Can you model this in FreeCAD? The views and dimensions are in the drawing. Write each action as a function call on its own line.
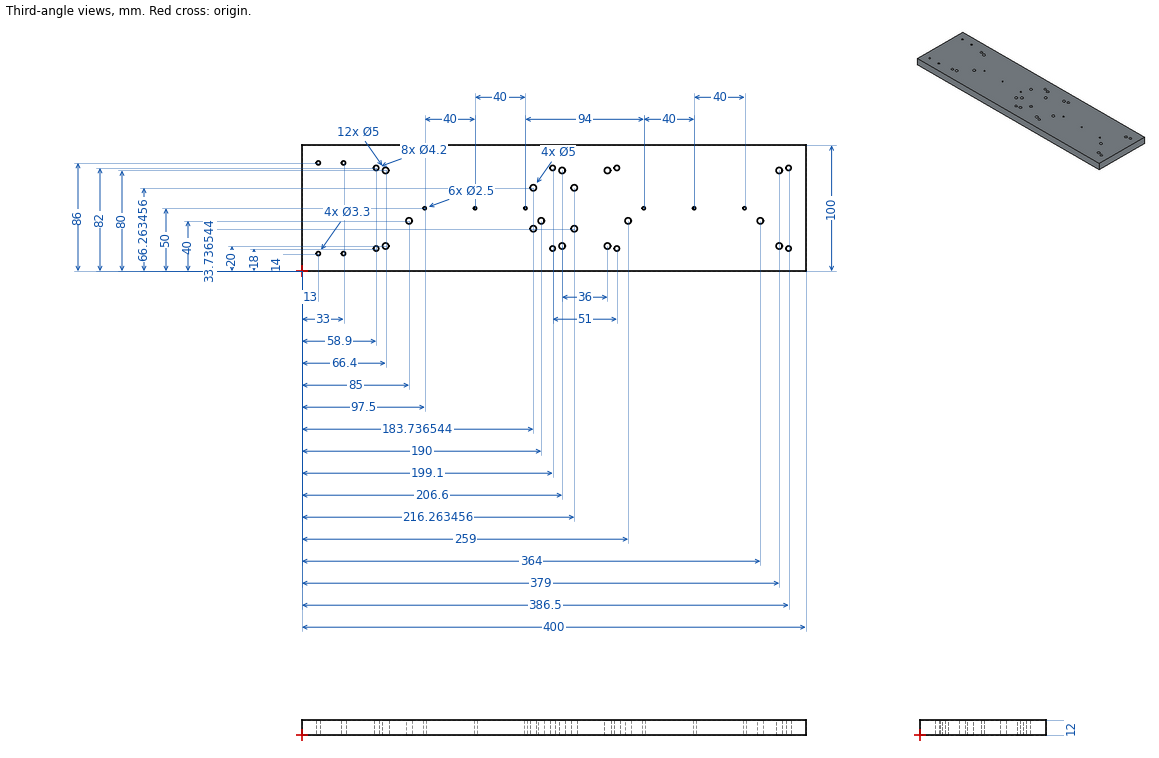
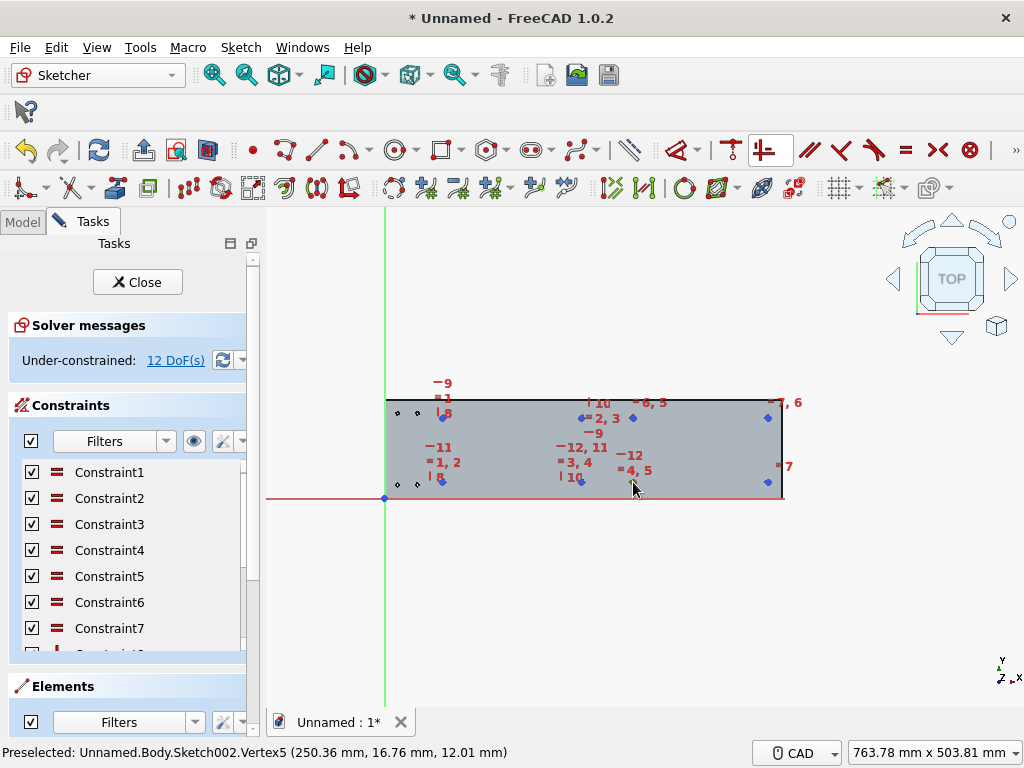
click(633, 418)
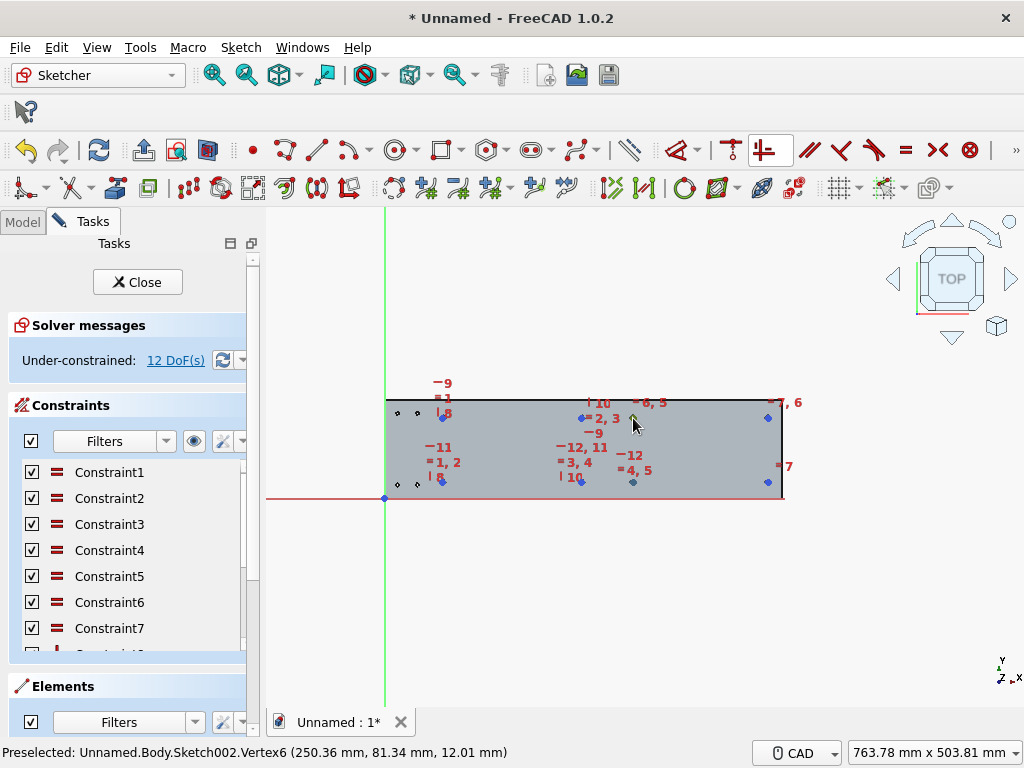
click(788, 150)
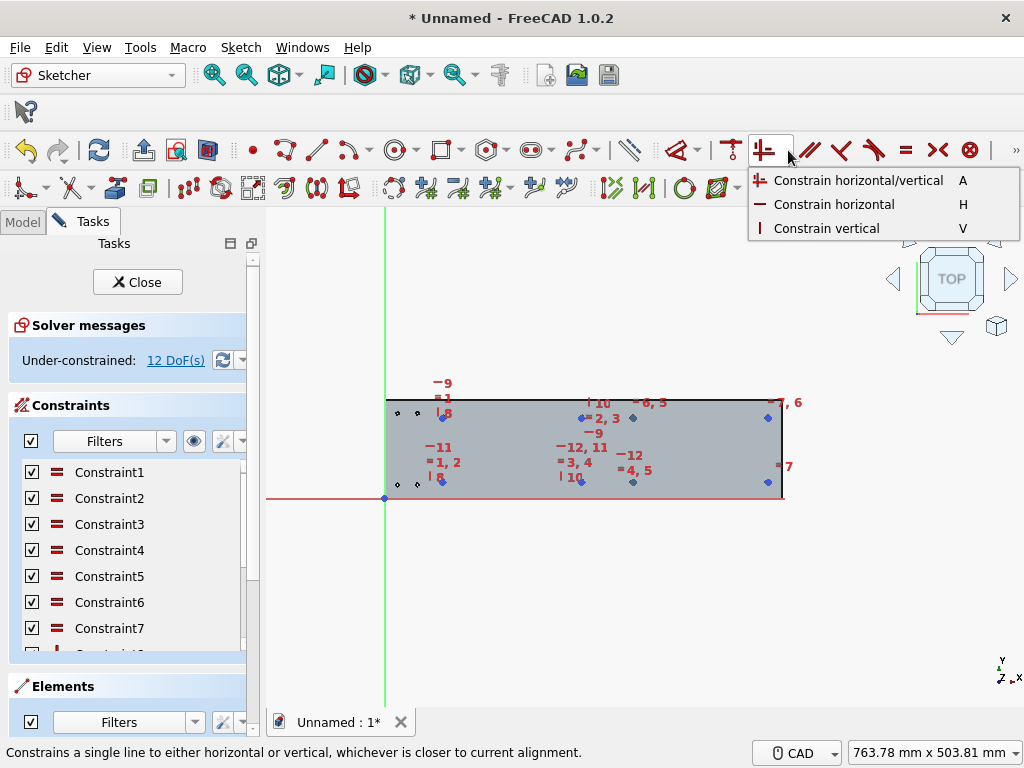
click(884, 228)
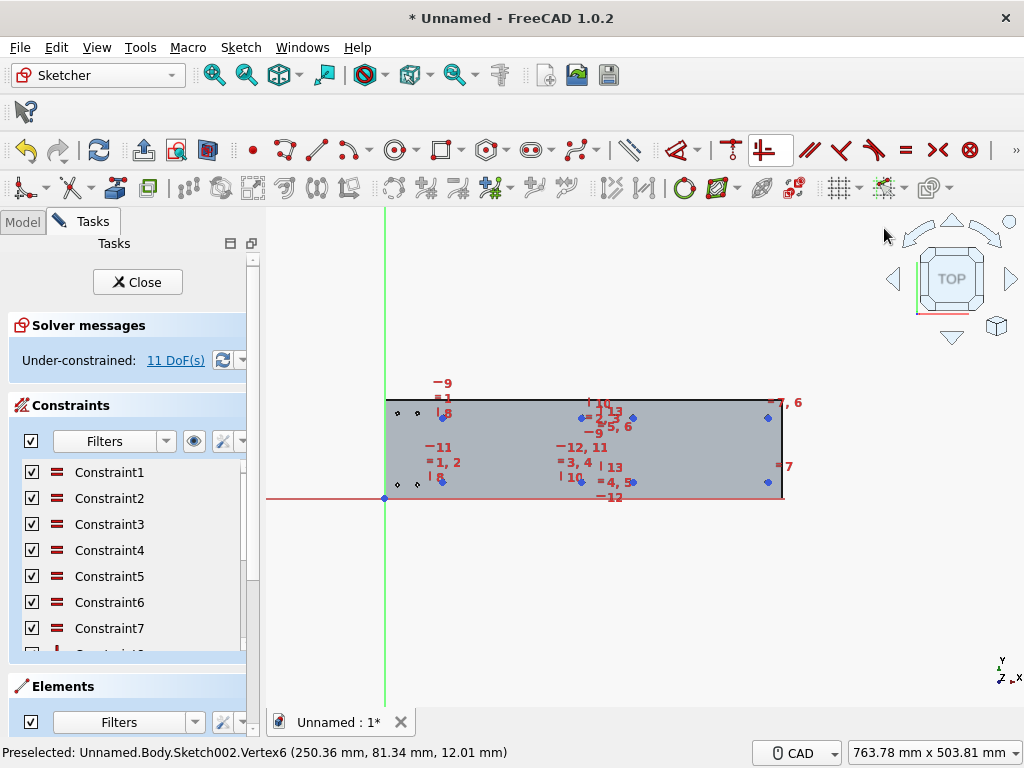
click(582, 418)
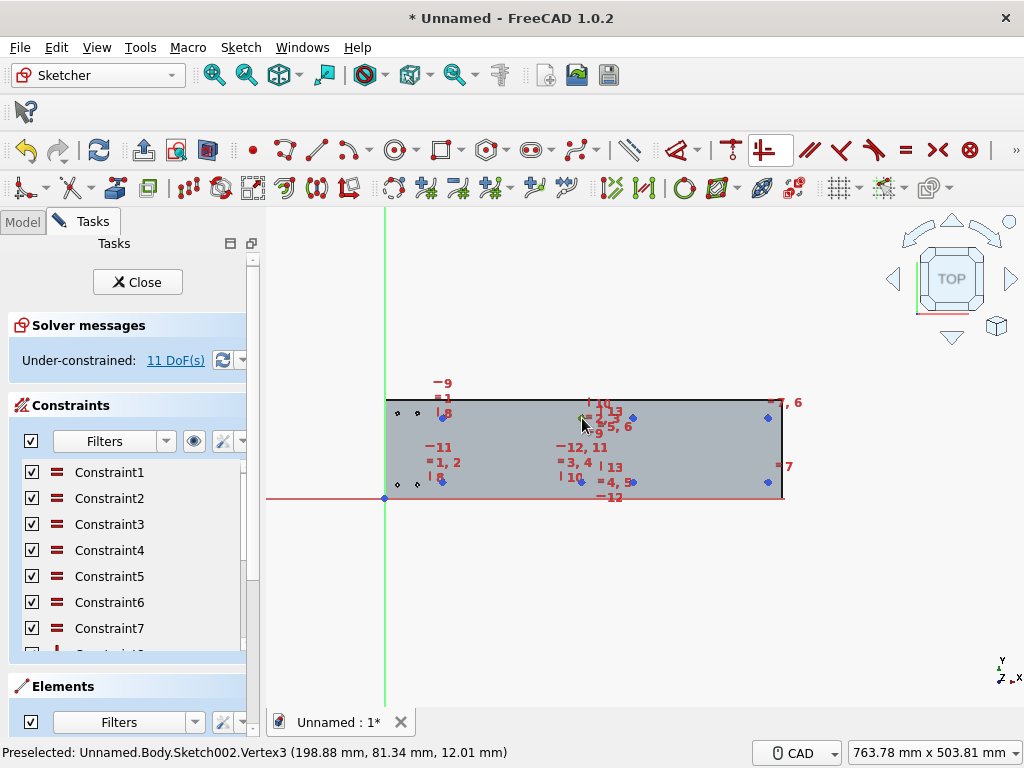
click(633, 418)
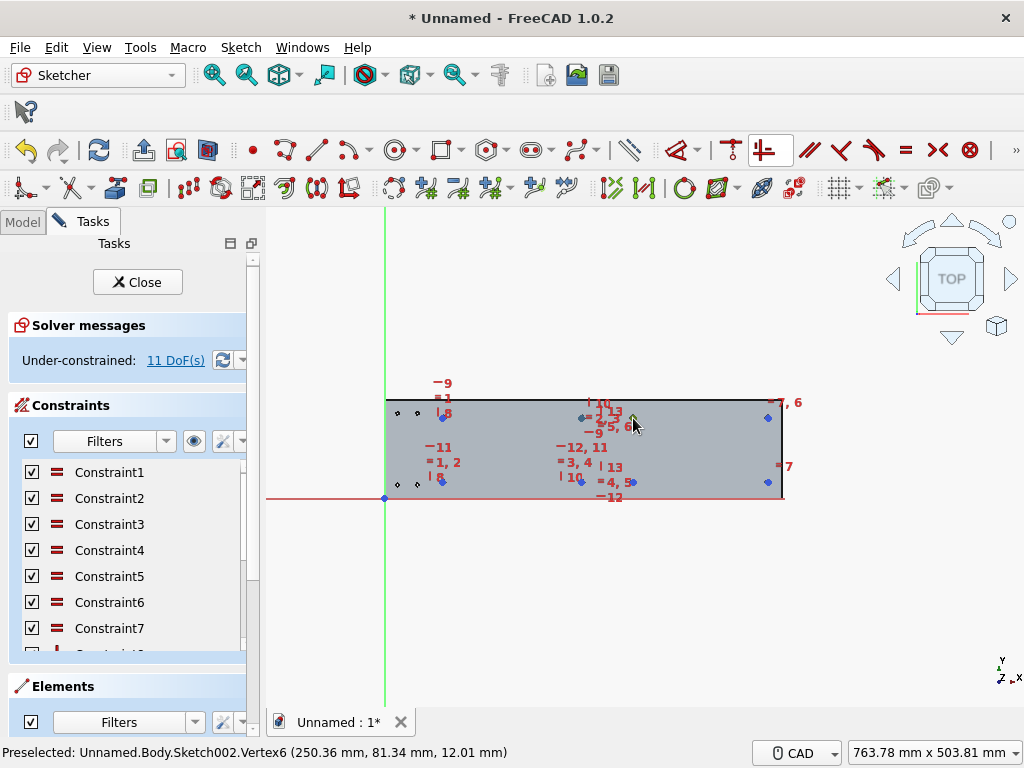
click(788, 150)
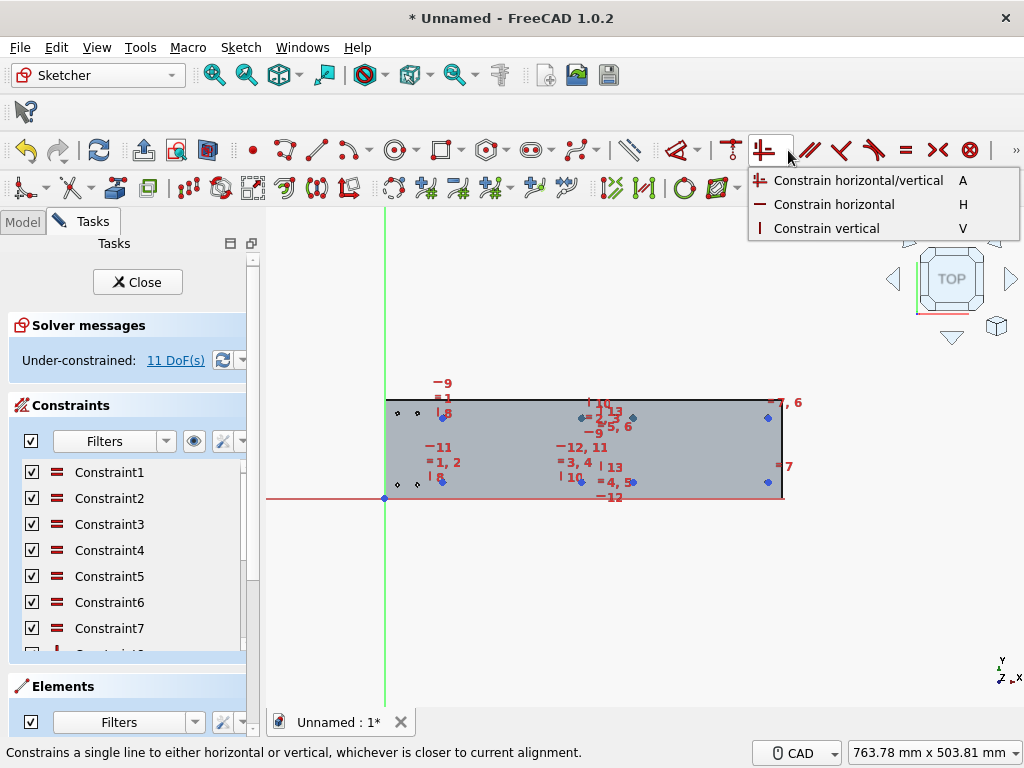
click(884, 204)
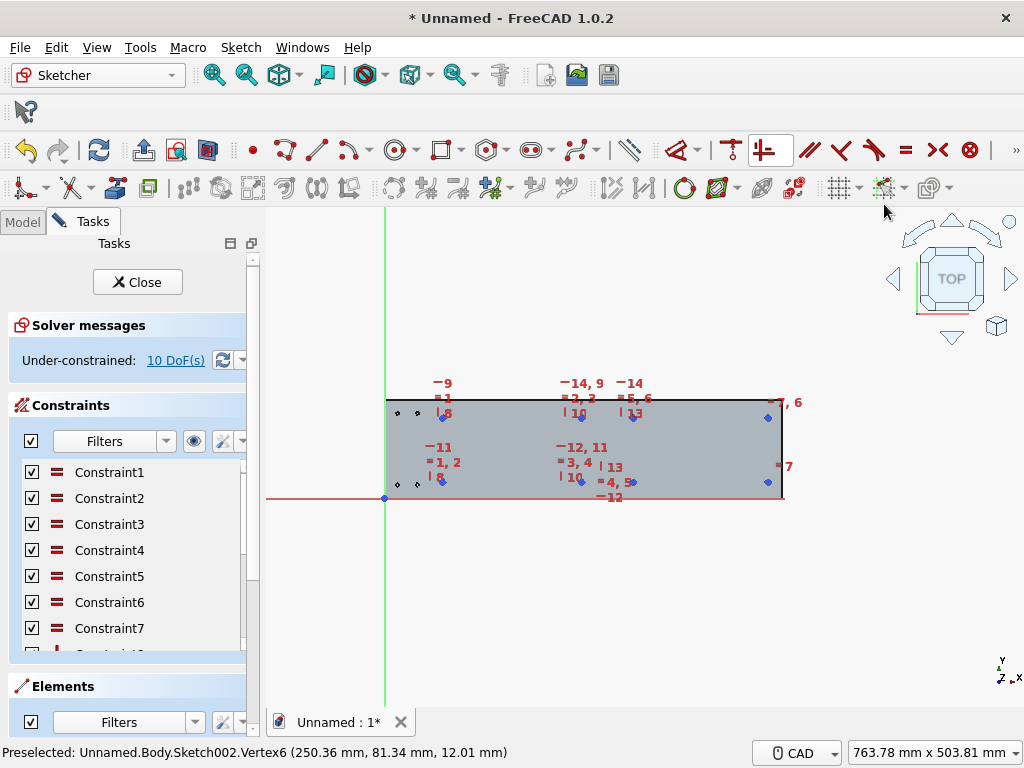
click(631, 420)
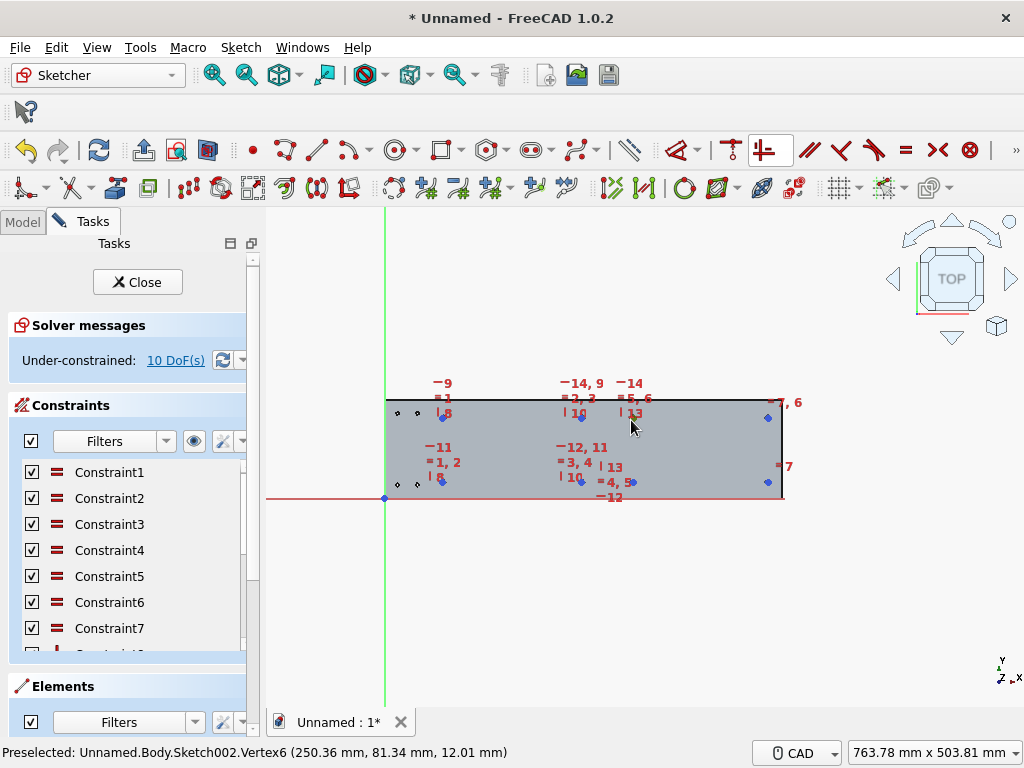
click(768, 418)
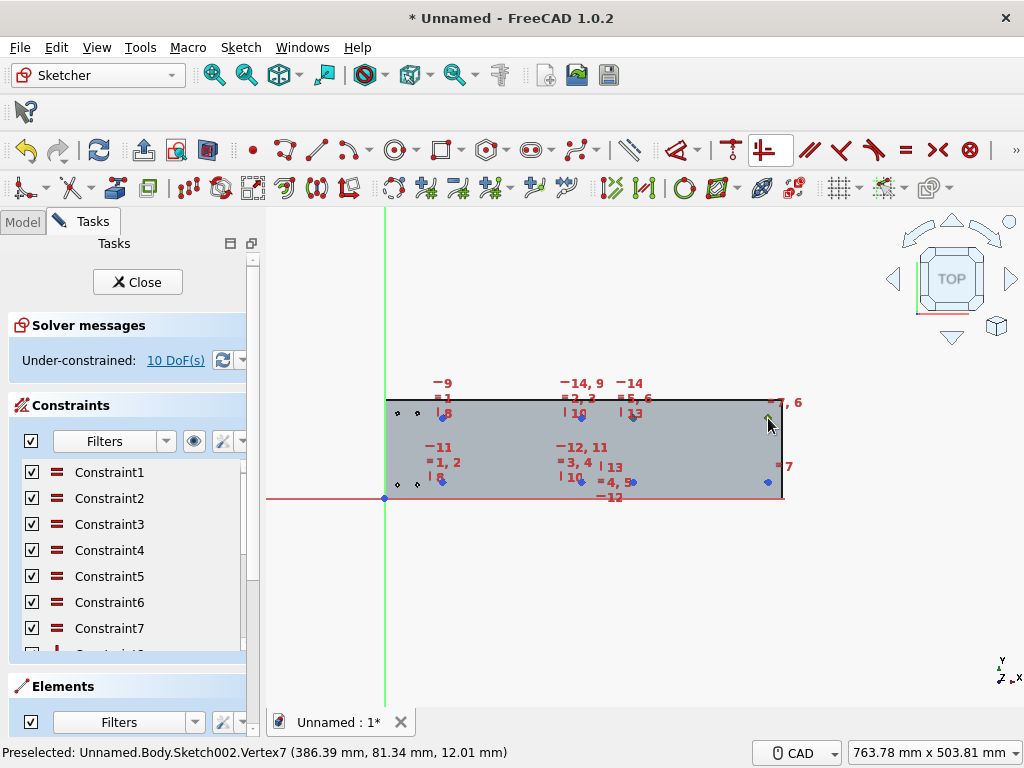
click(788, 150)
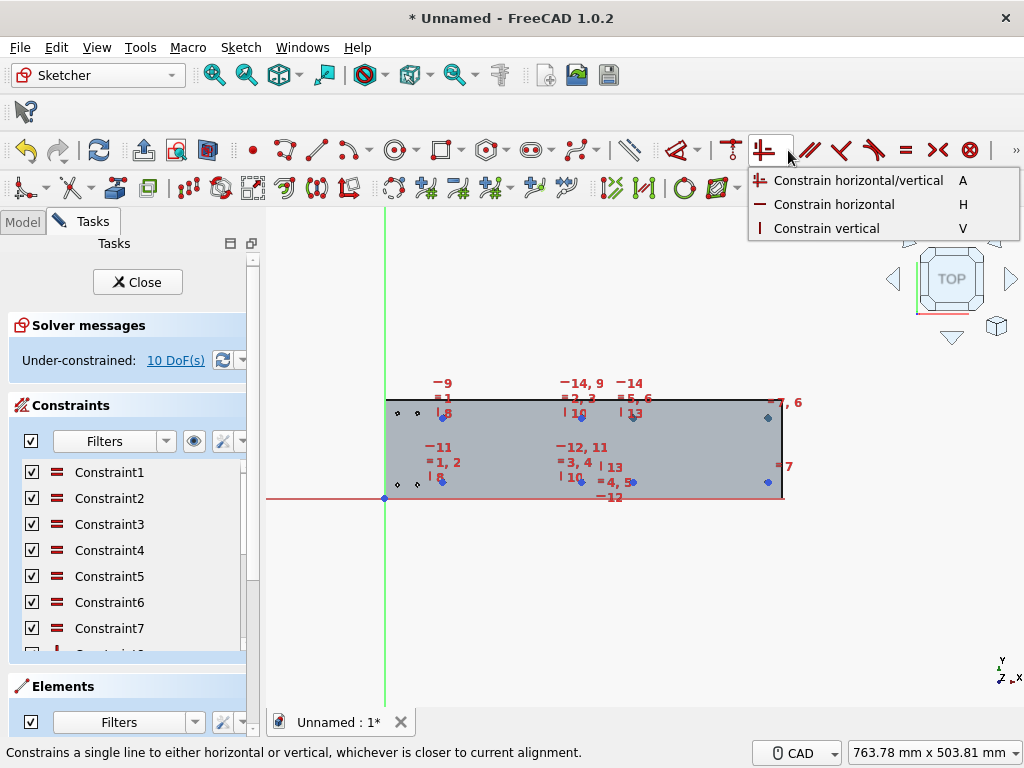
click(884, 204)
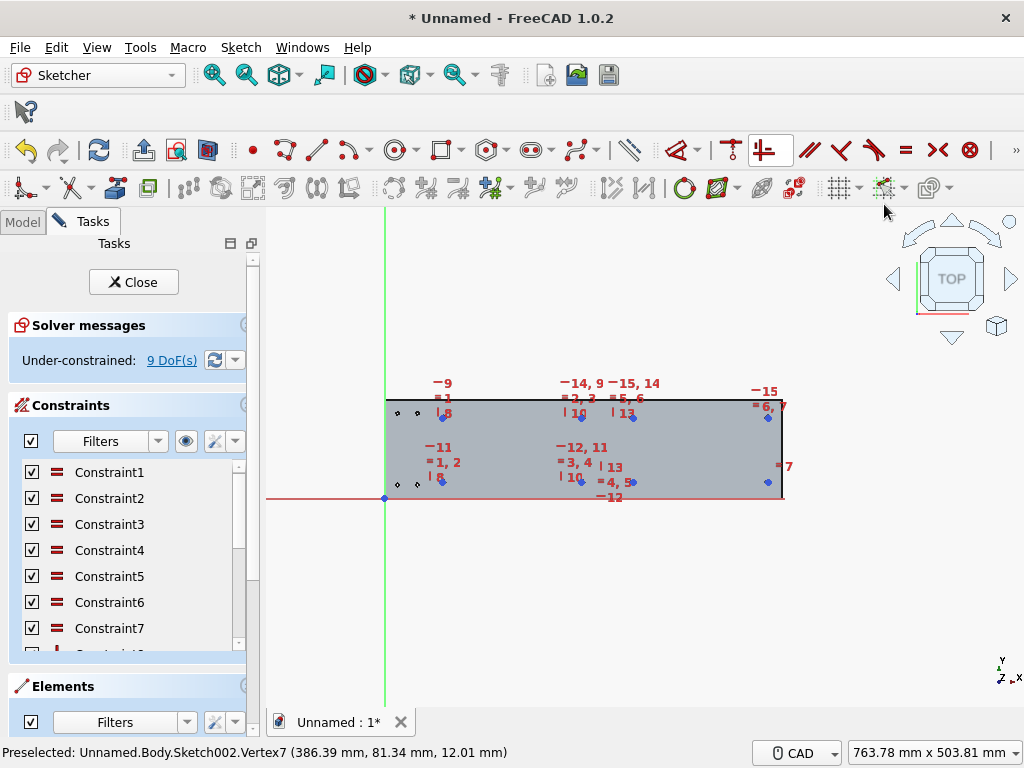
click(768, 418)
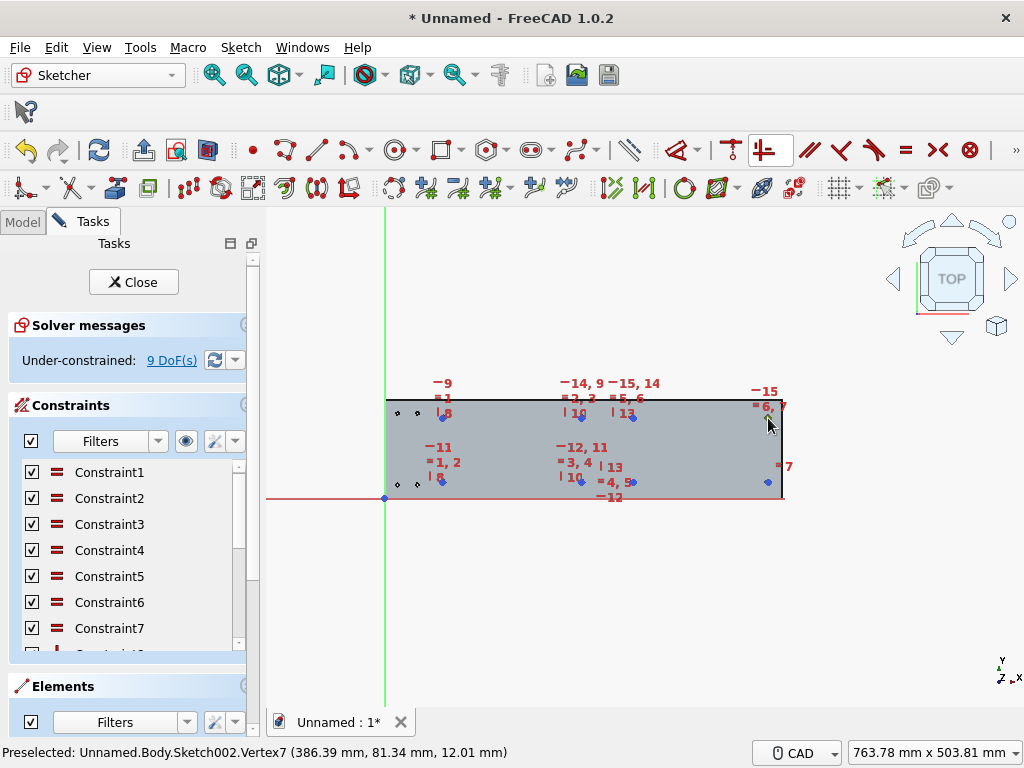
click(768, 482)